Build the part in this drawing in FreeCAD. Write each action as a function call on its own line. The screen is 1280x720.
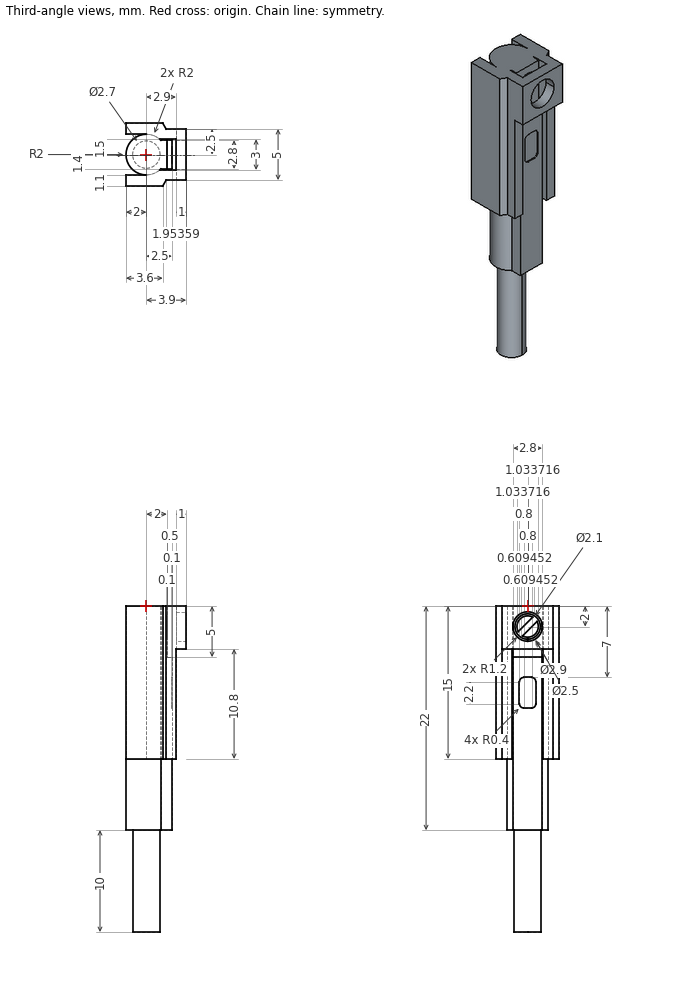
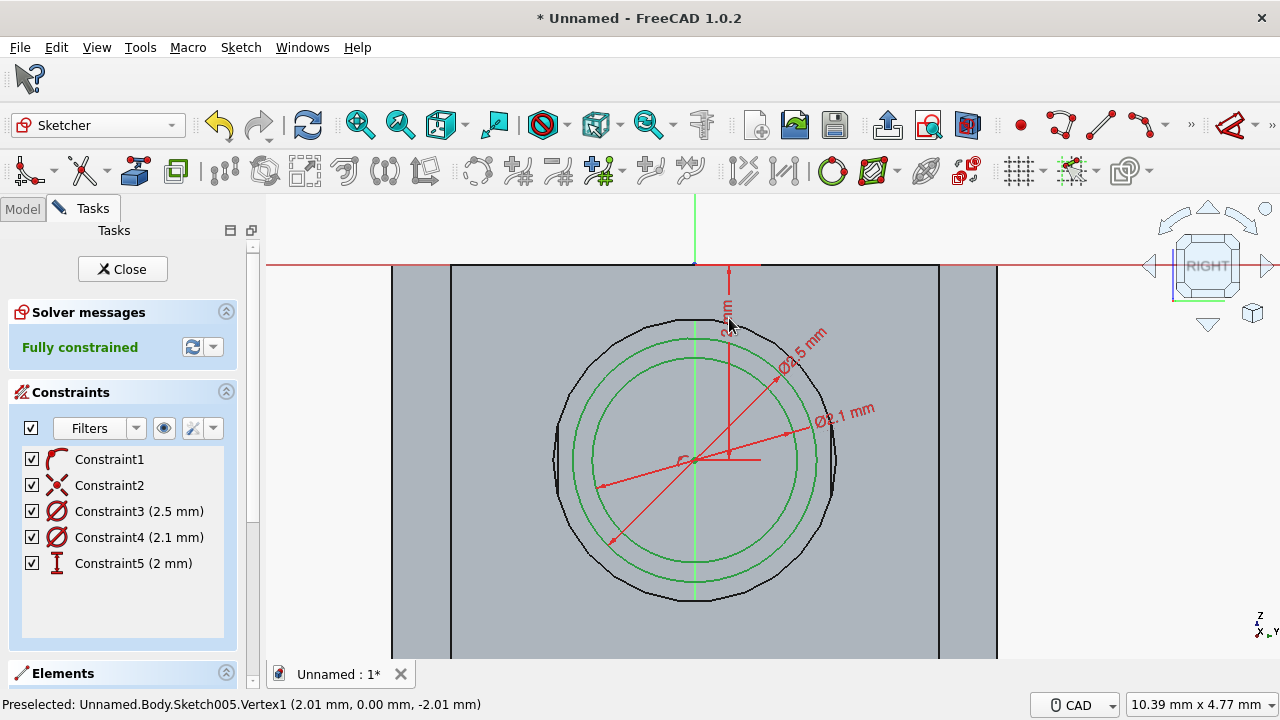
click(123, 269)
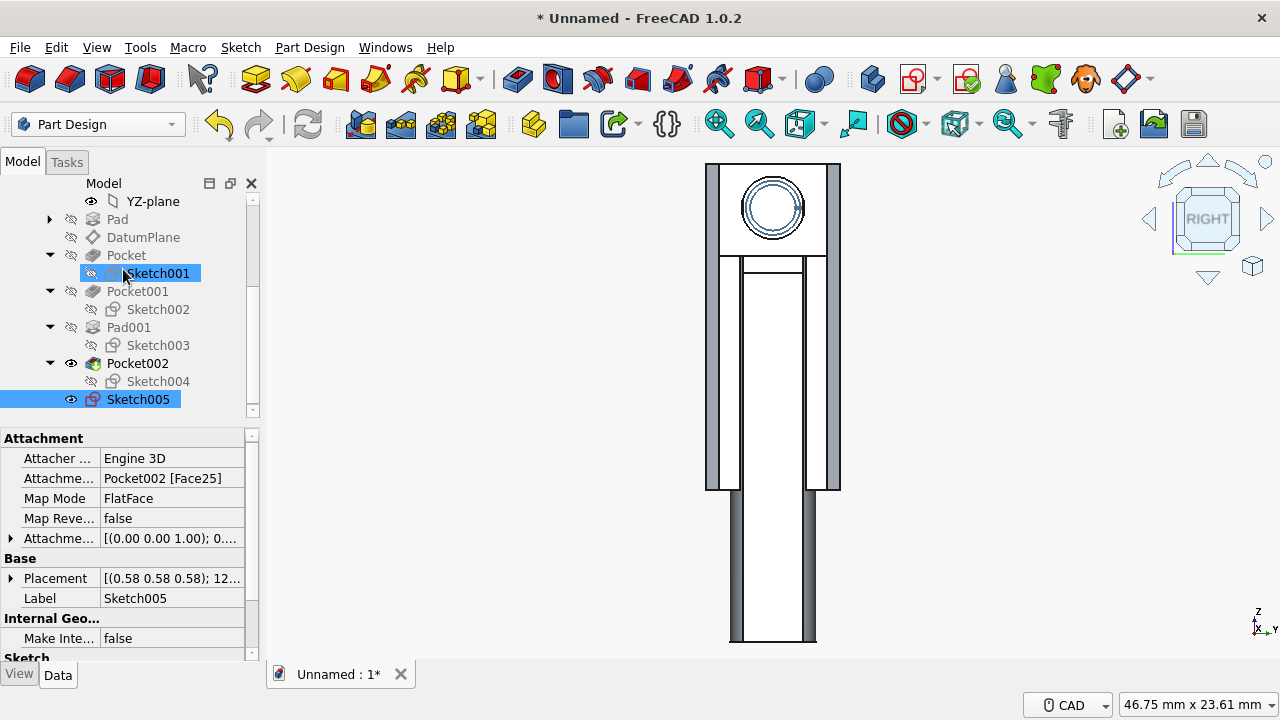
click(518, 80)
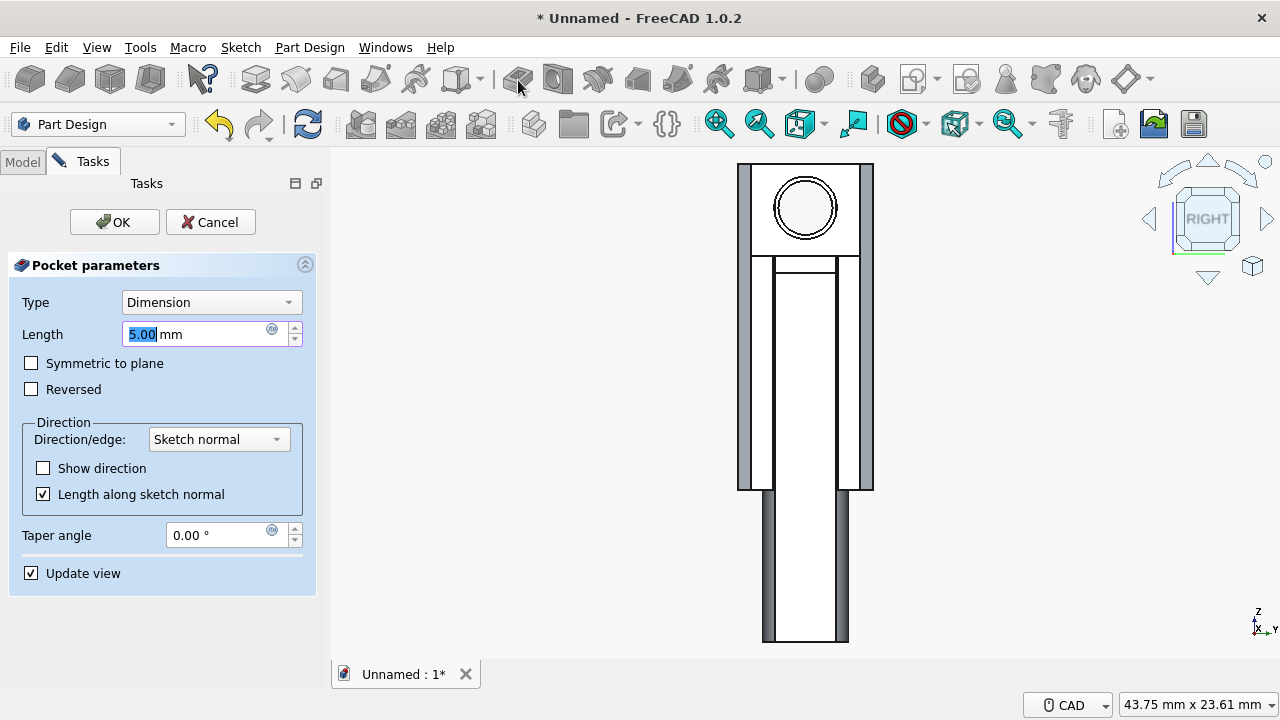
text(0.1)
key(Tab)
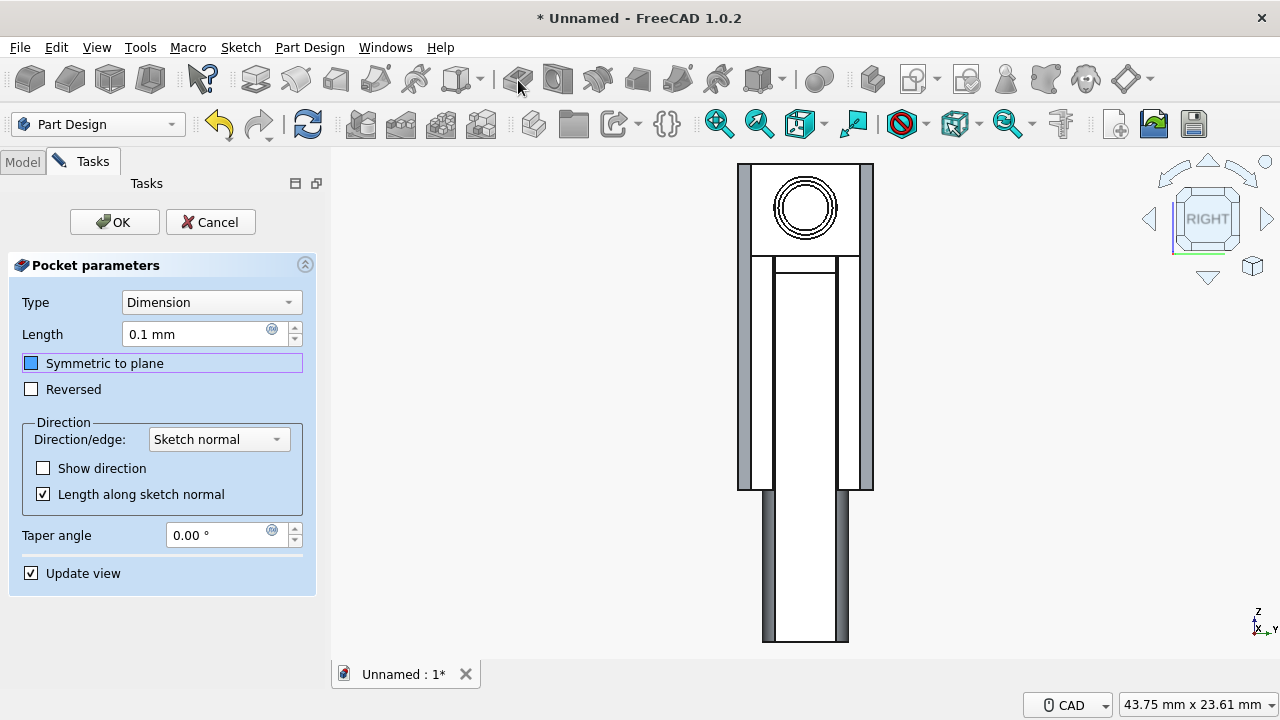
click(115, 222)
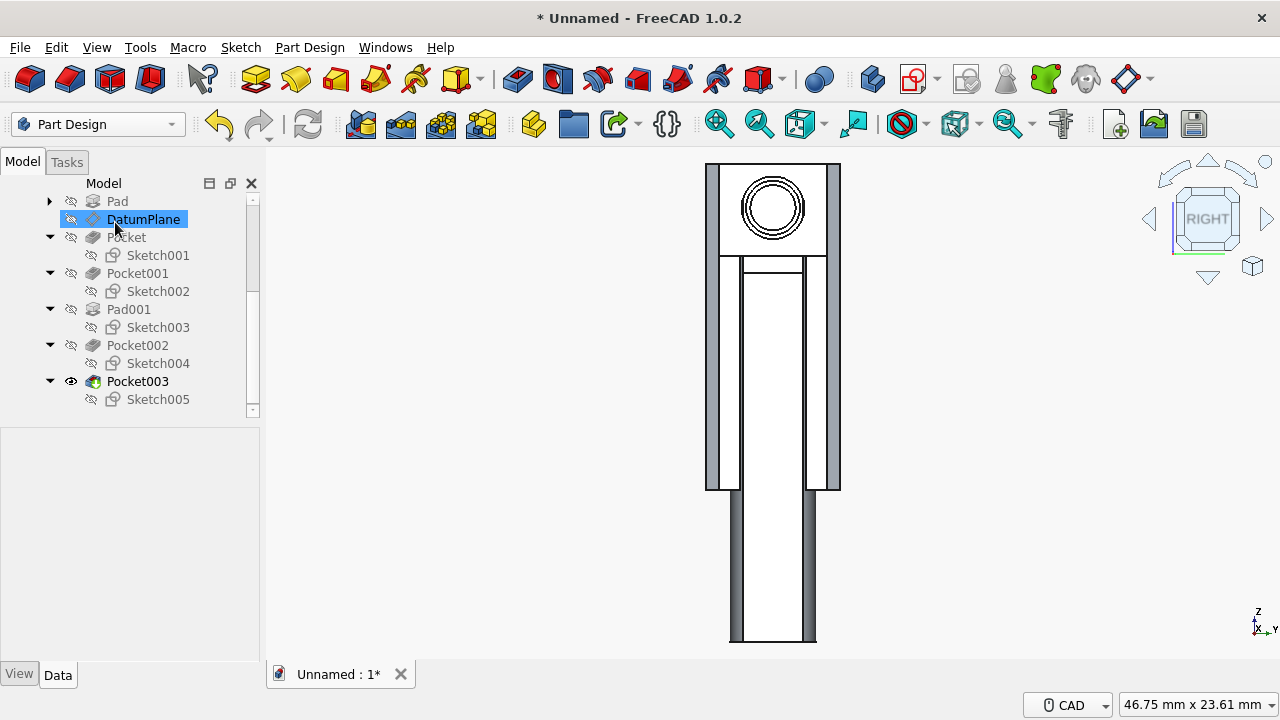
click(773, 207)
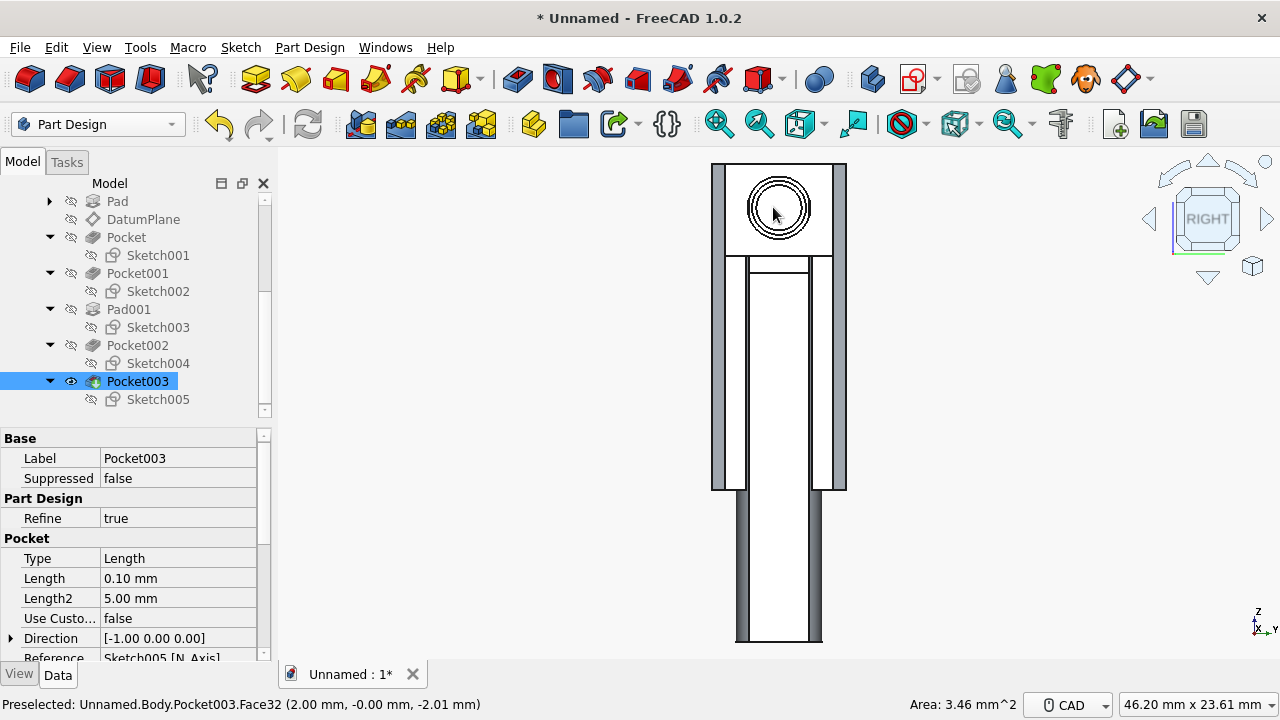
click(914, 80)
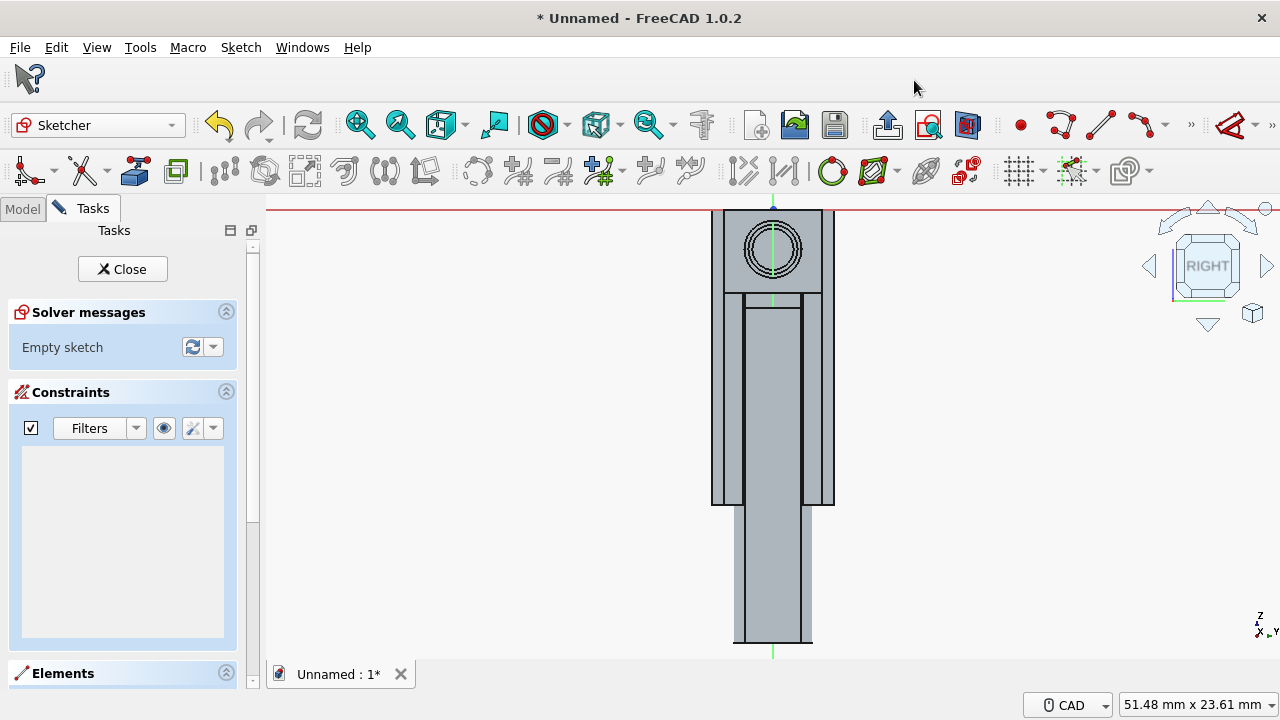
click(968, 126)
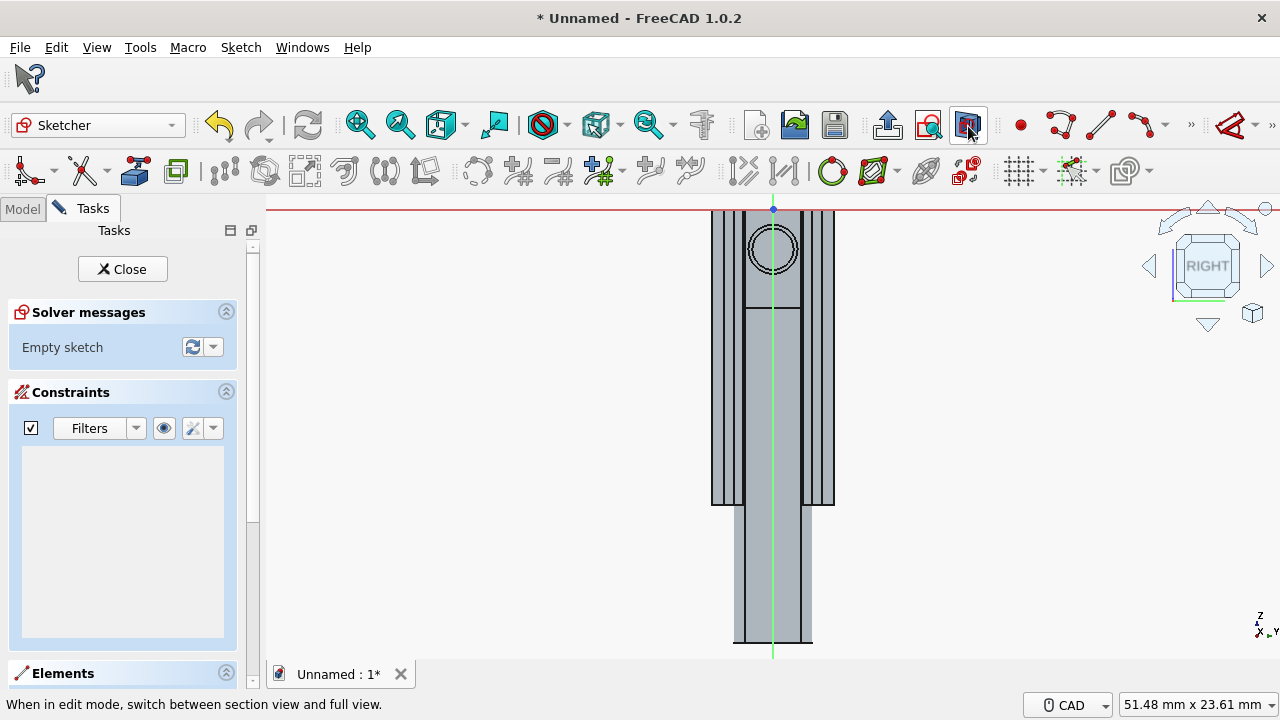
scroll(704, 426, down, 5)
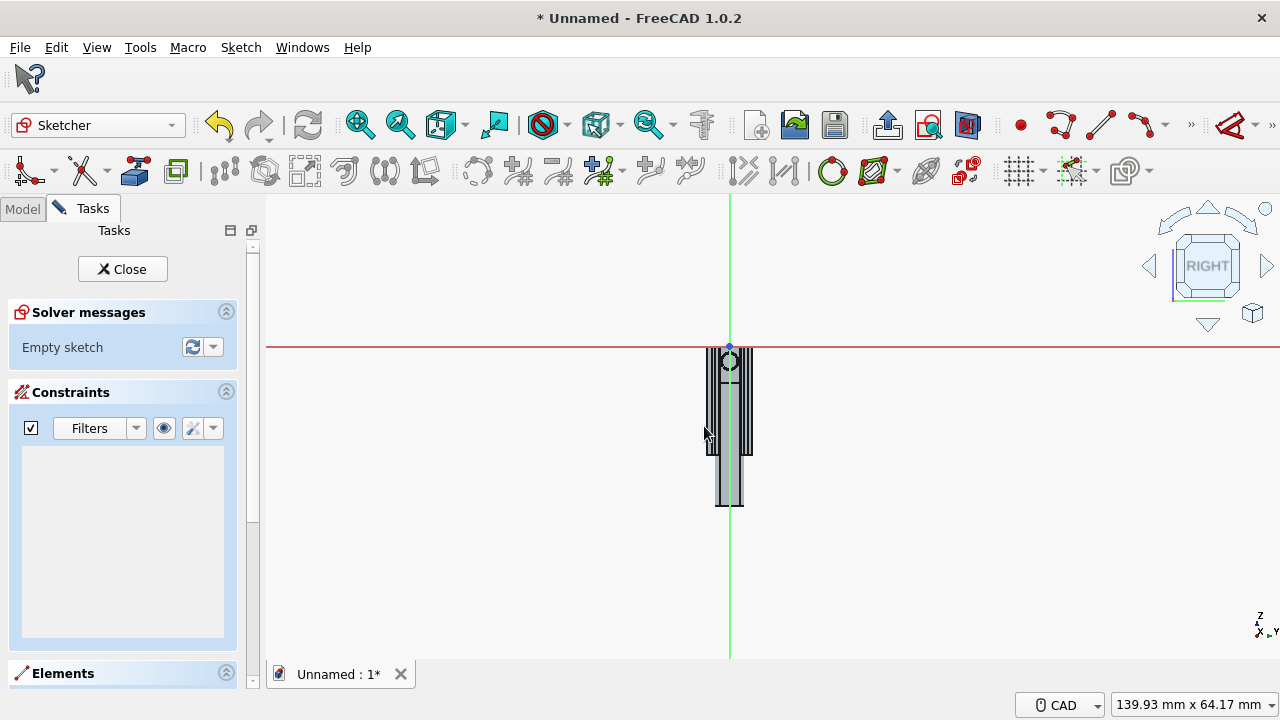
scroll(732, 352, up, 13)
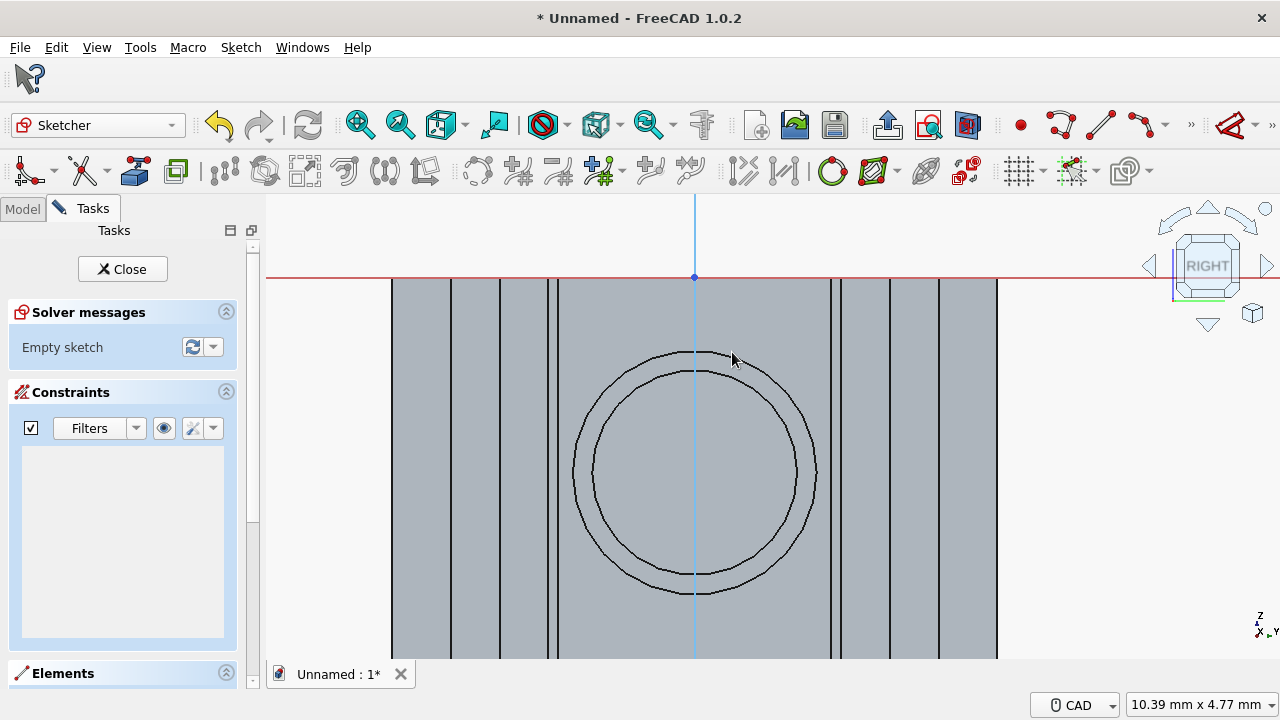
click(1102, 126)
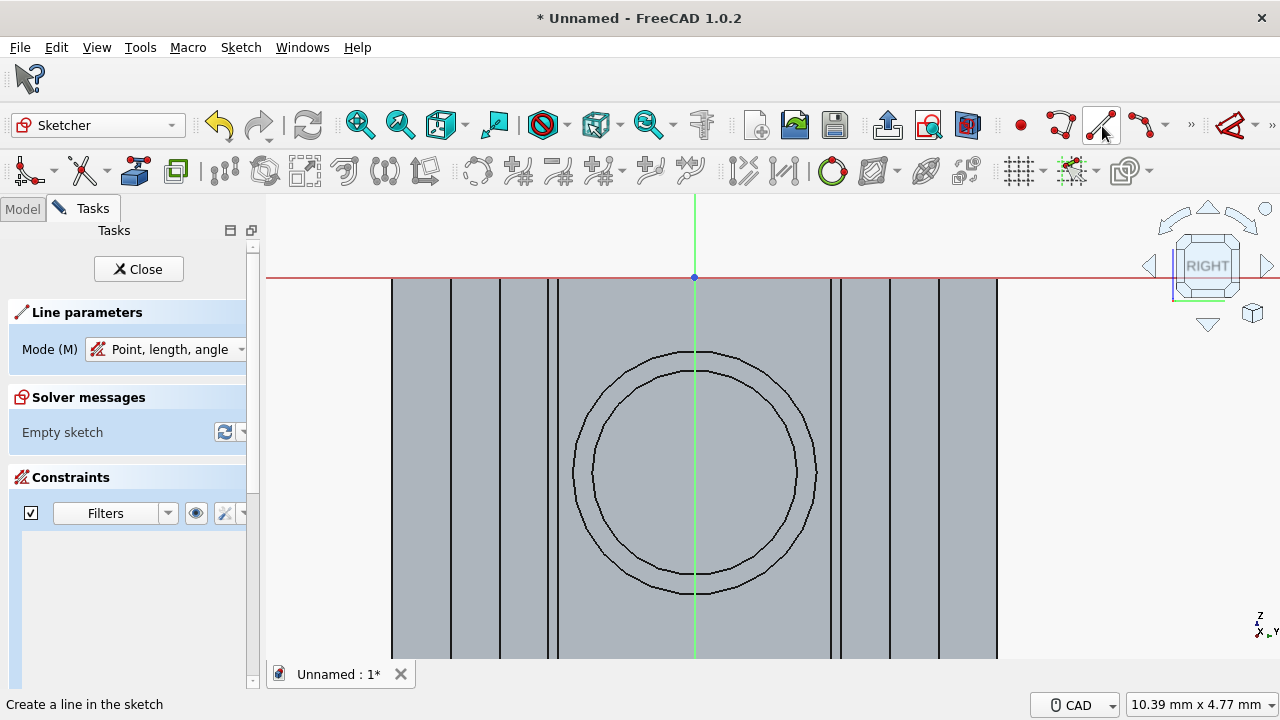
click(754, 372)
click(594, 532)